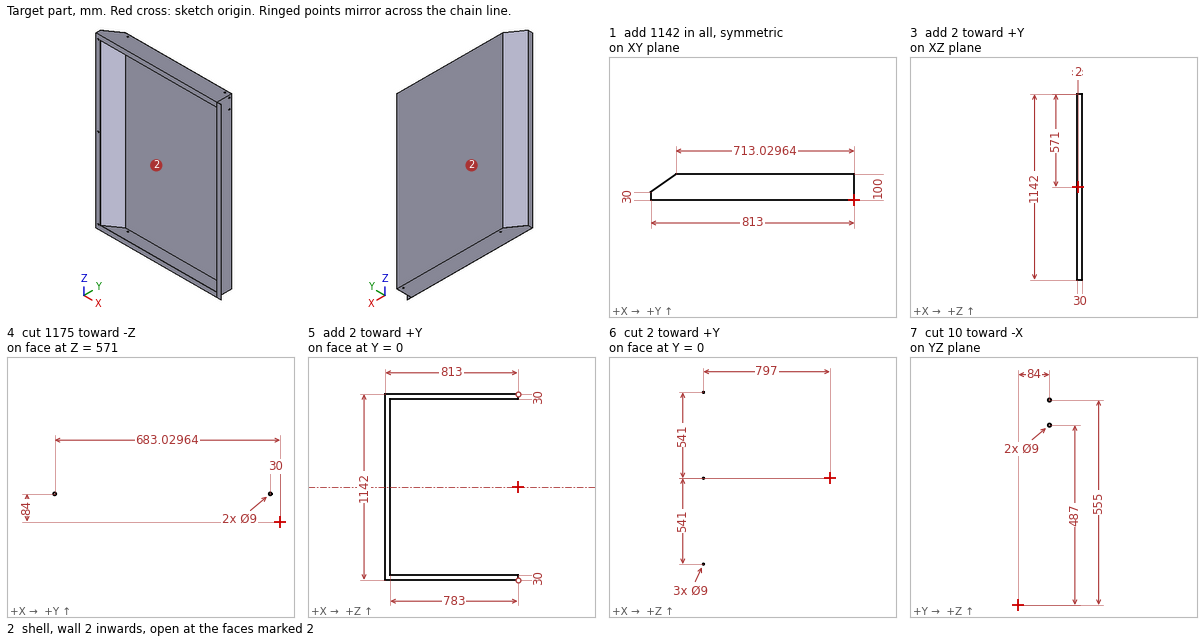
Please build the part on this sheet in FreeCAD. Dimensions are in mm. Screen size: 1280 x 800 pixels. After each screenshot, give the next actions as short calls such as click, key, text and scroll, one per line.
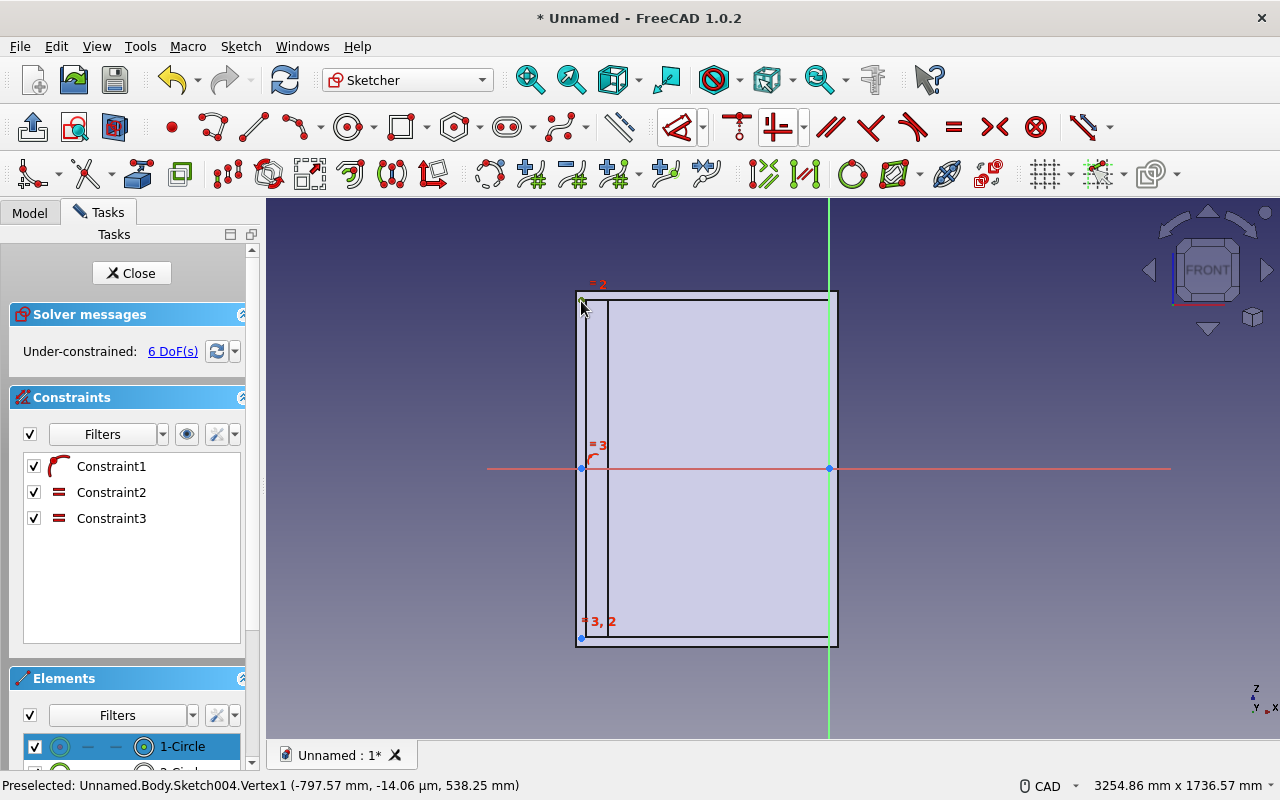
click(581, 638)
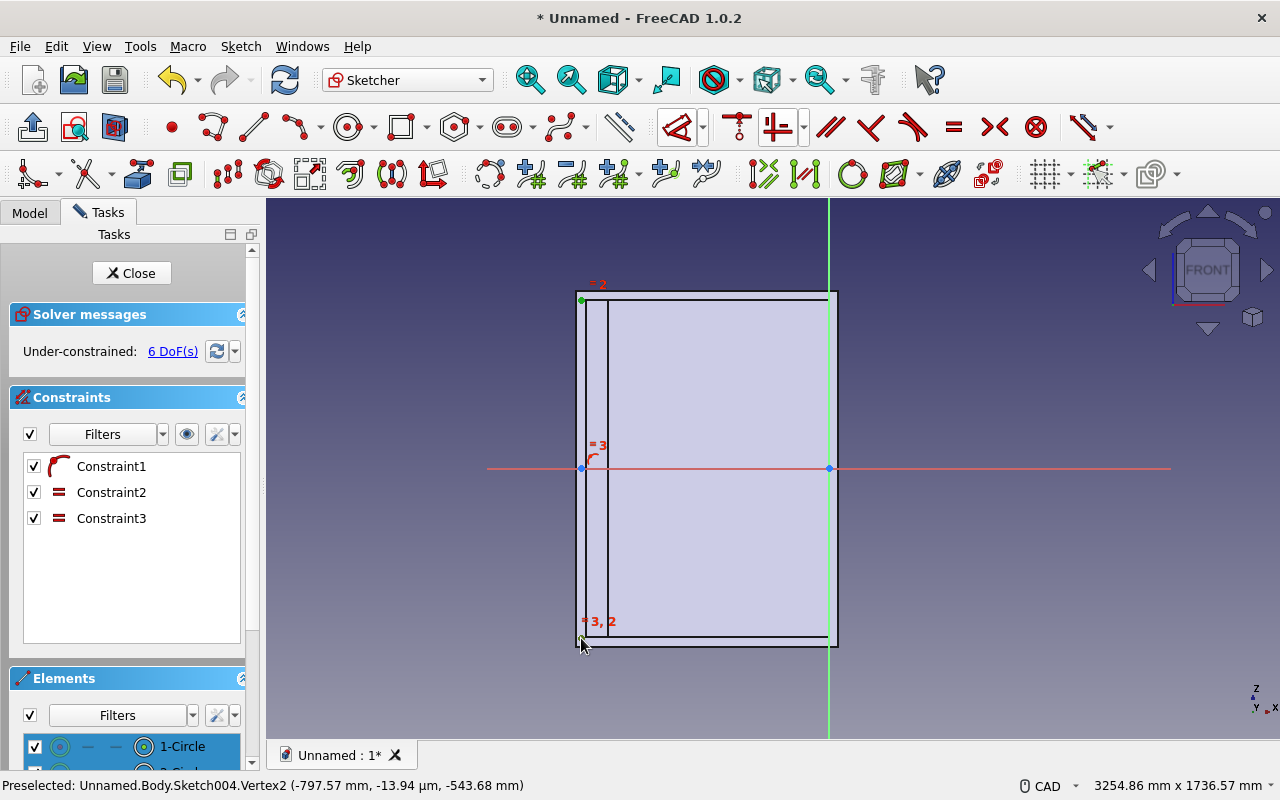
key(v)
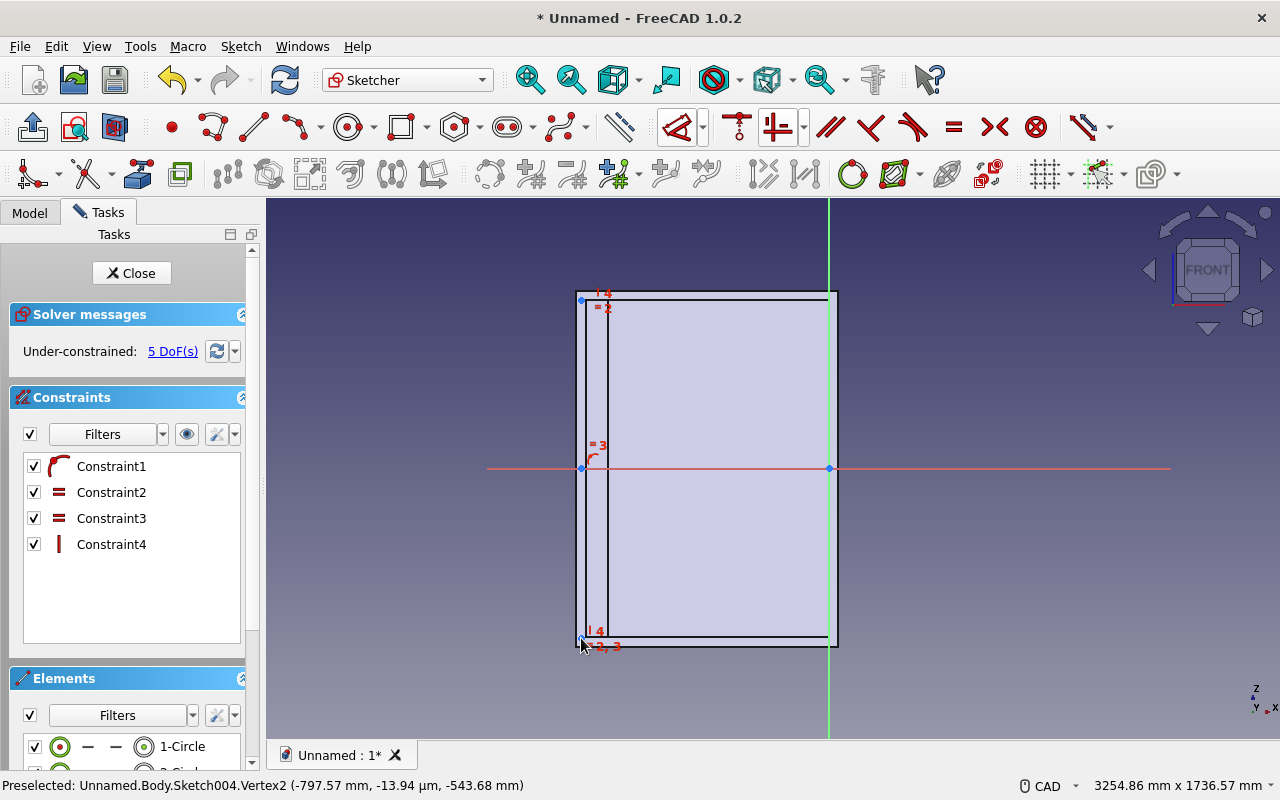
click(581, 301)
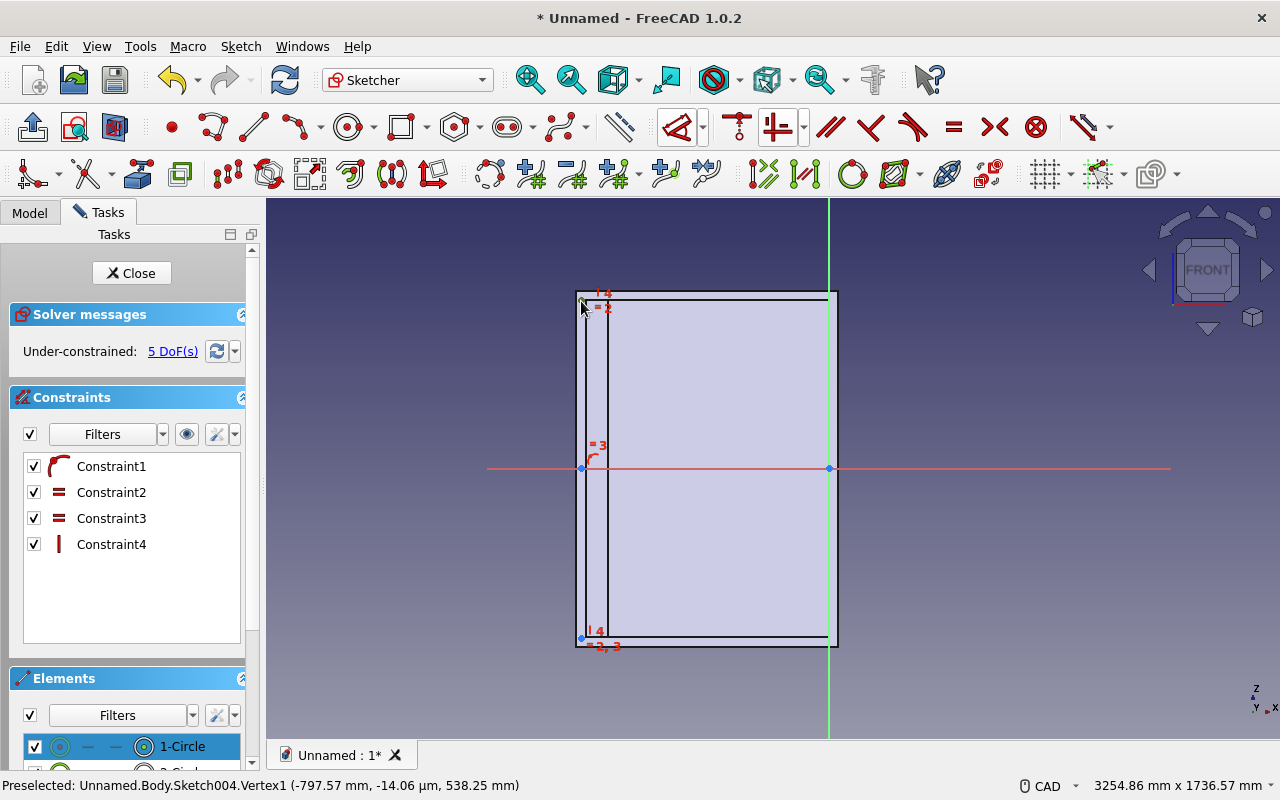
click(581, 469)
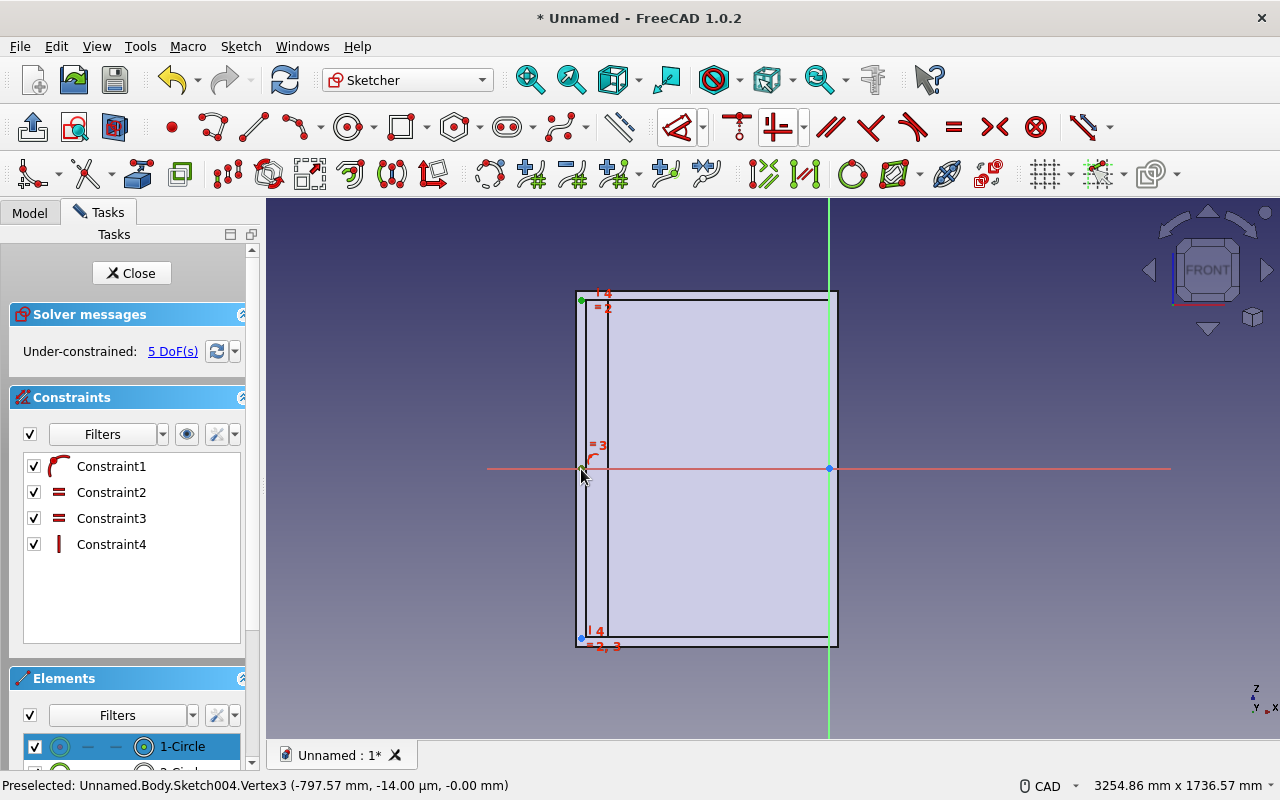
key(v)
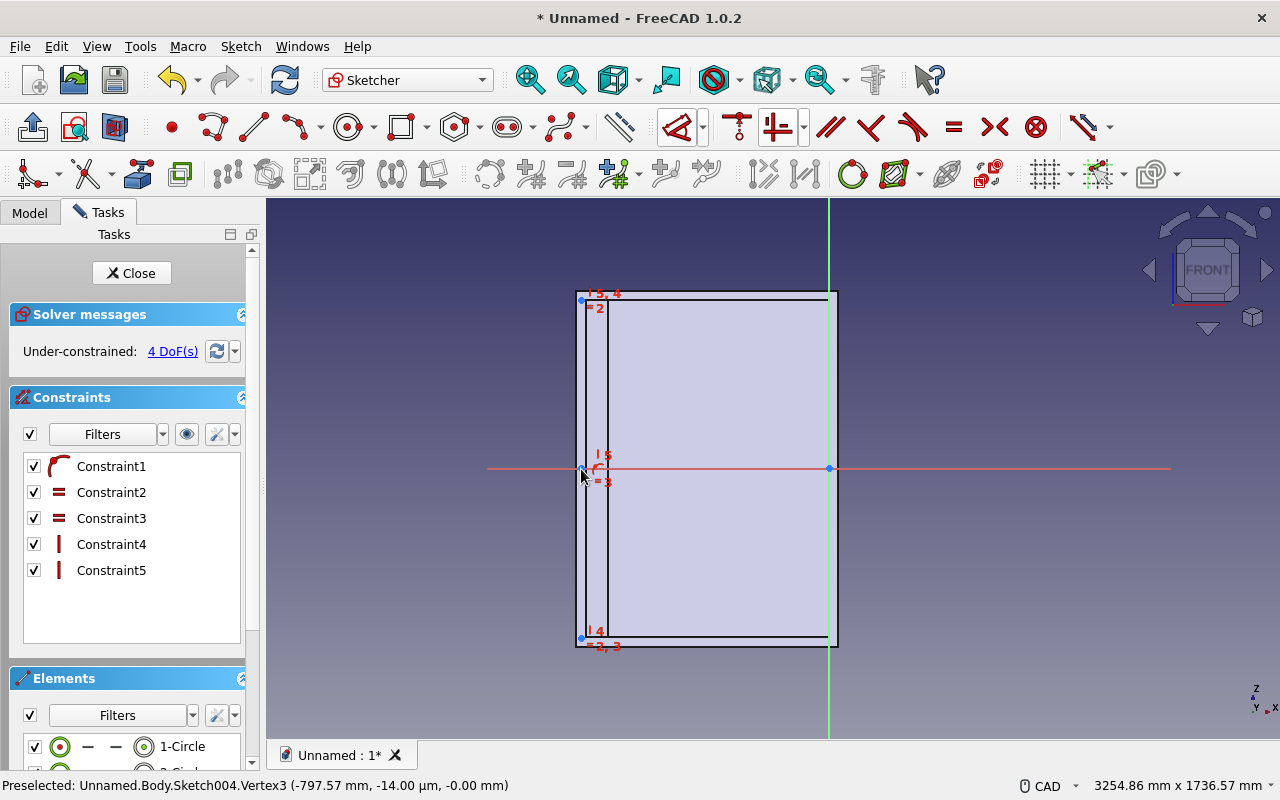
scroll(581, 299, up, 14)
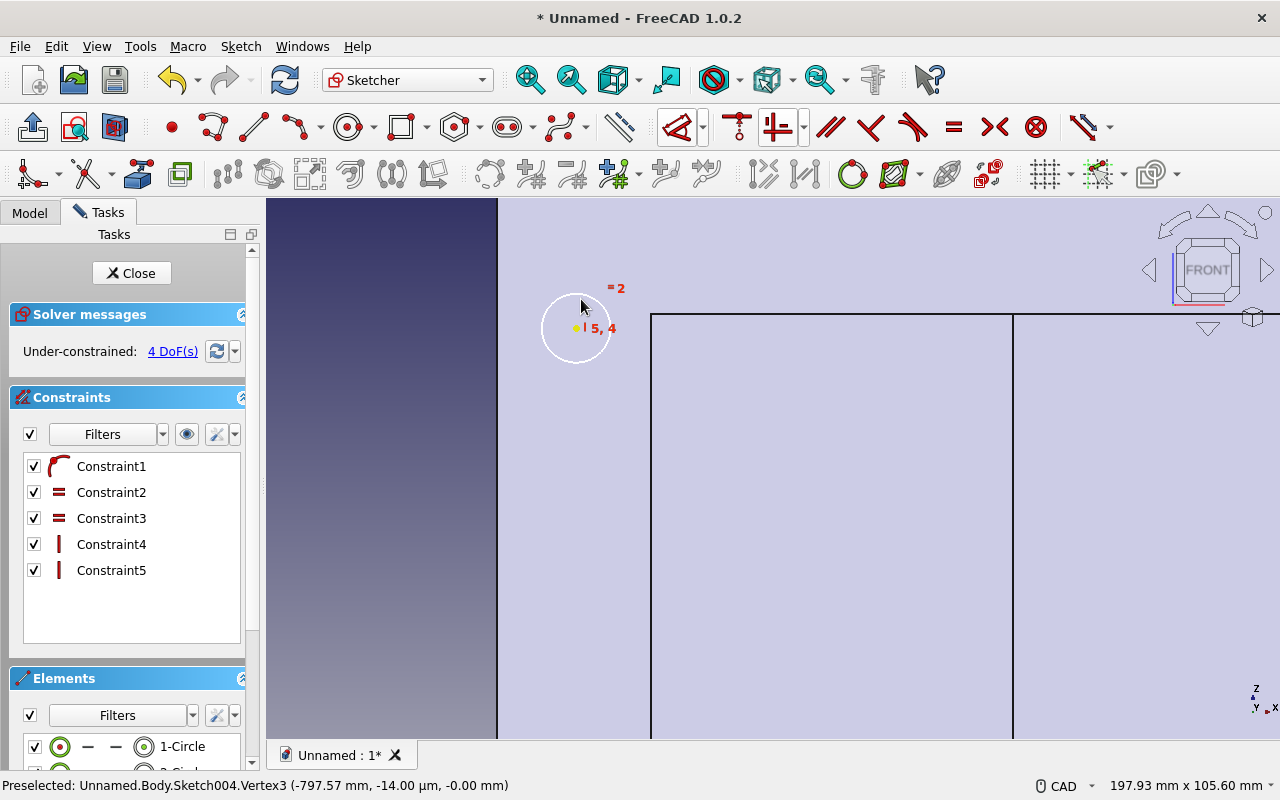
click(577, 294)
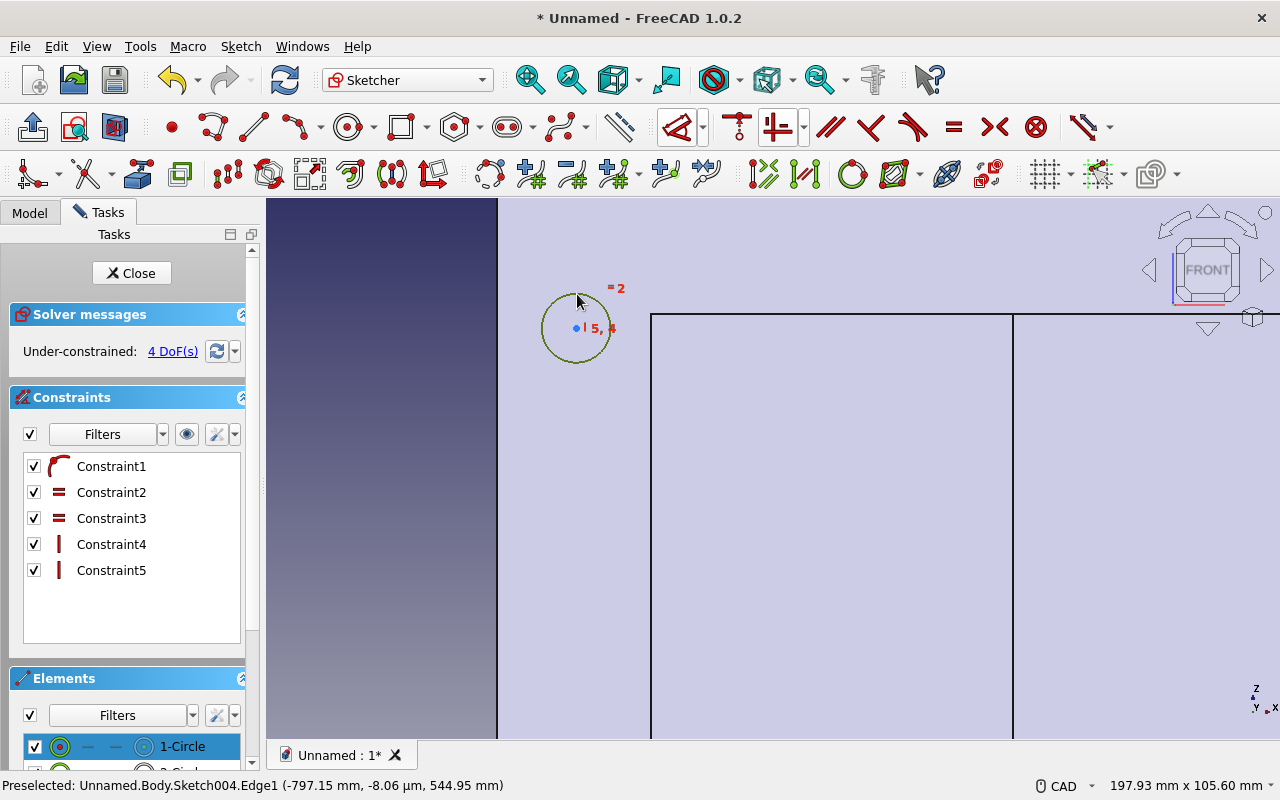
key(k)
key(o)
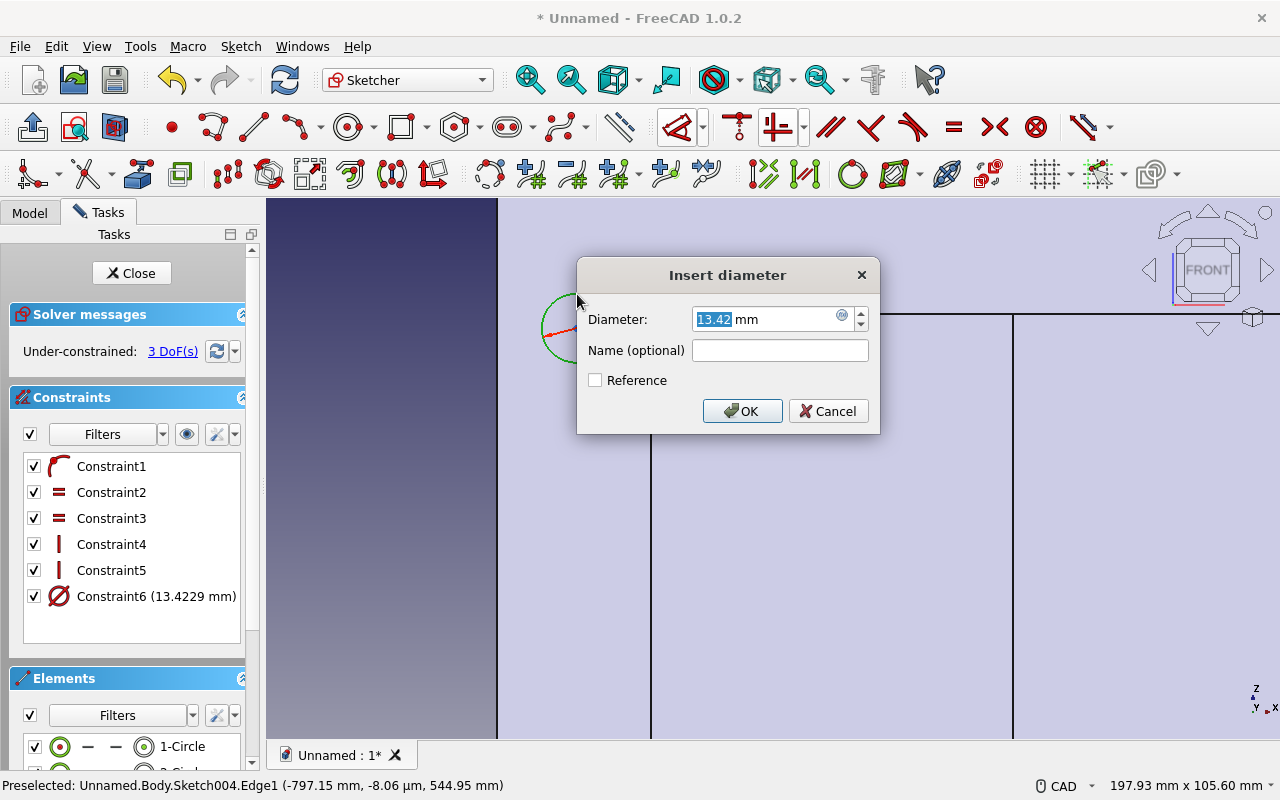
text(9)
key(Return)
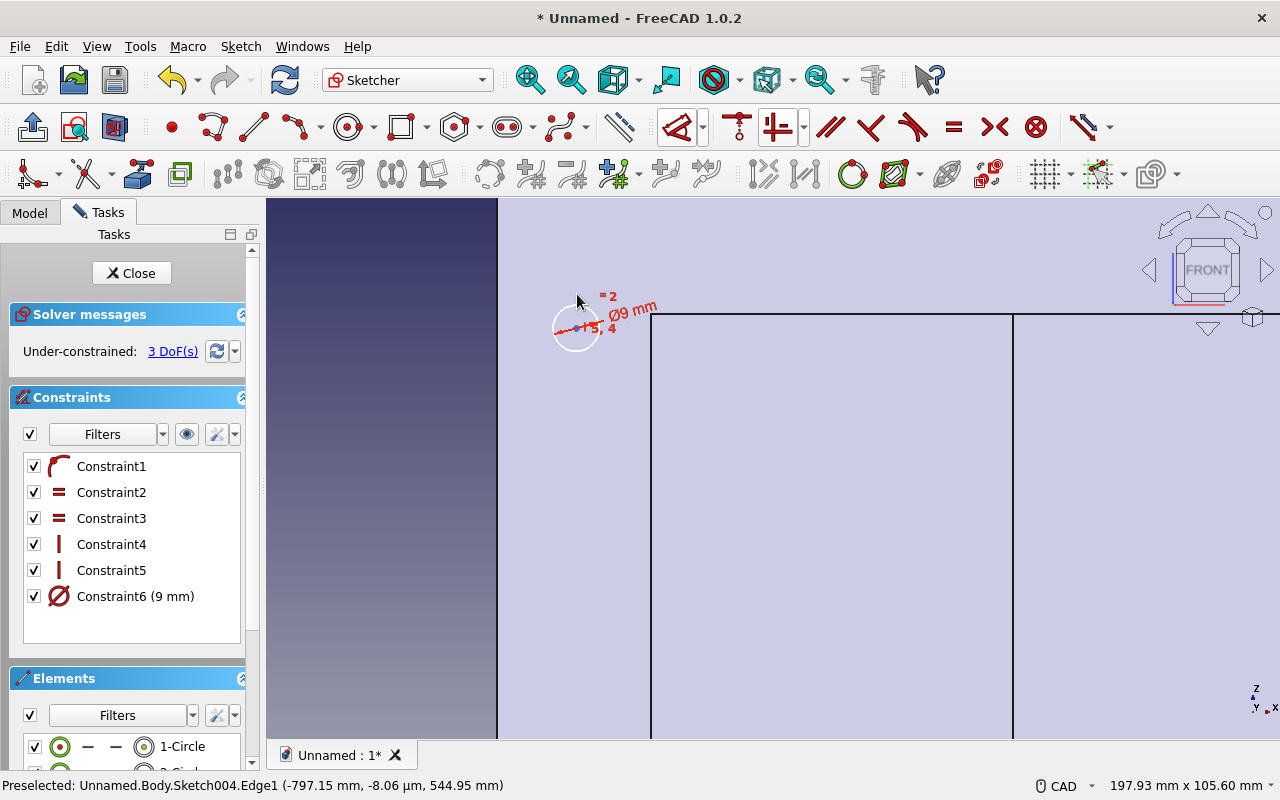
scroll(581, 299, down, 14)